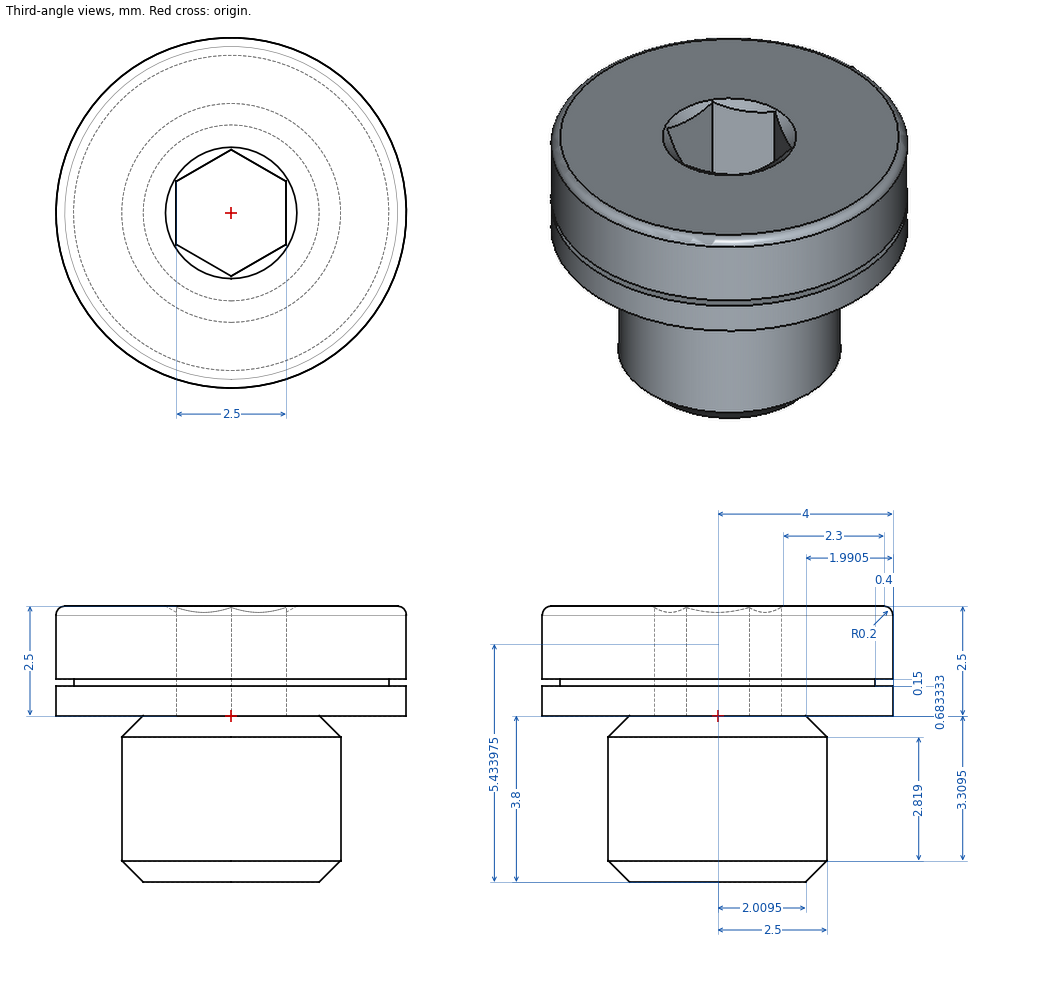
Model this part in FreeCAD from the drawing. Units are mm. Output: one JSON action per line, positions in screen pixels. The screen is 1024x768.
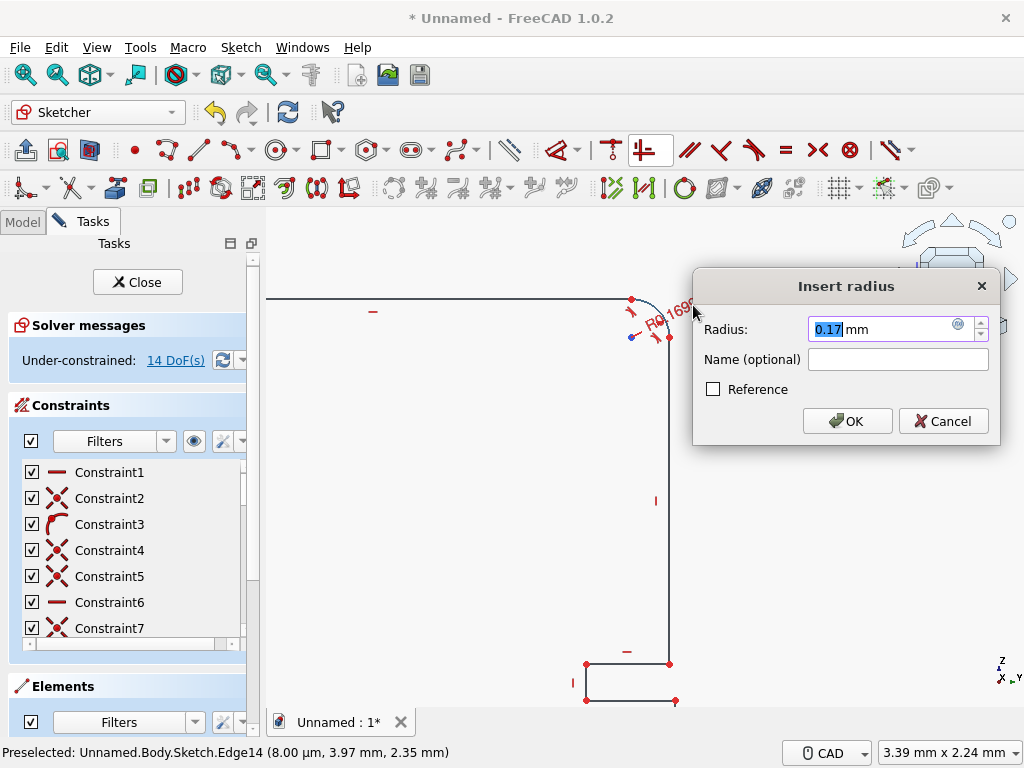
{"action": "type", "text": "0.2"}
{"action": "key", "text": "Return"}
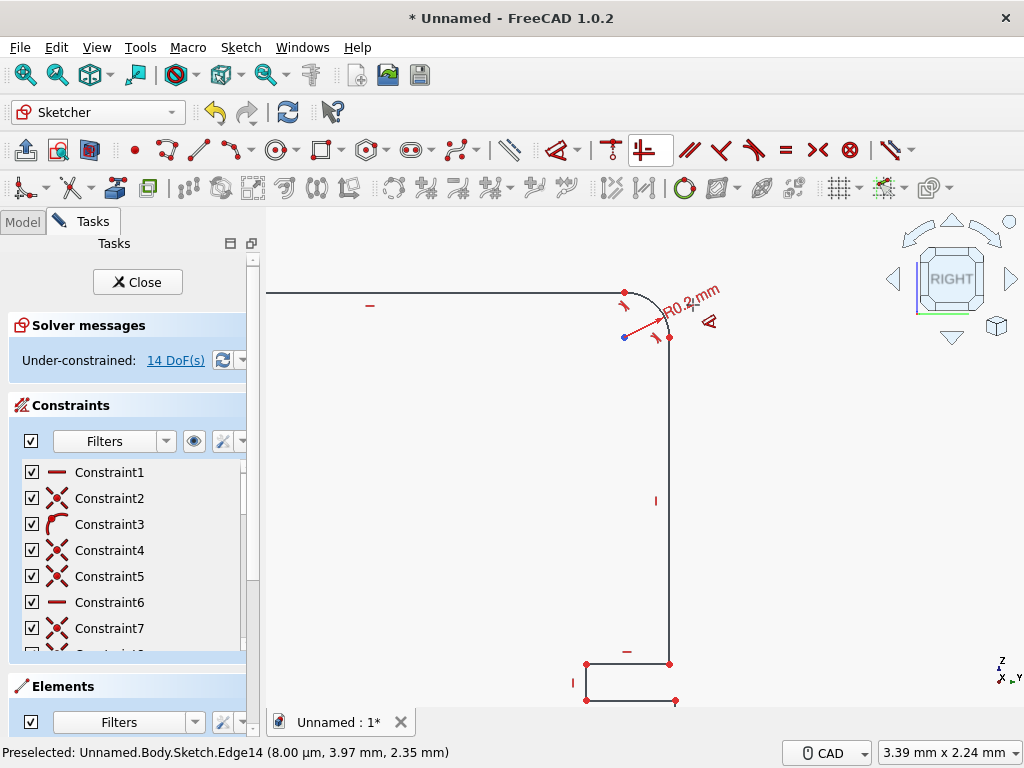
{"action": "scroll", "coordinate": [665, 321], "scroll_direction": "down", "scroll_amount": 8}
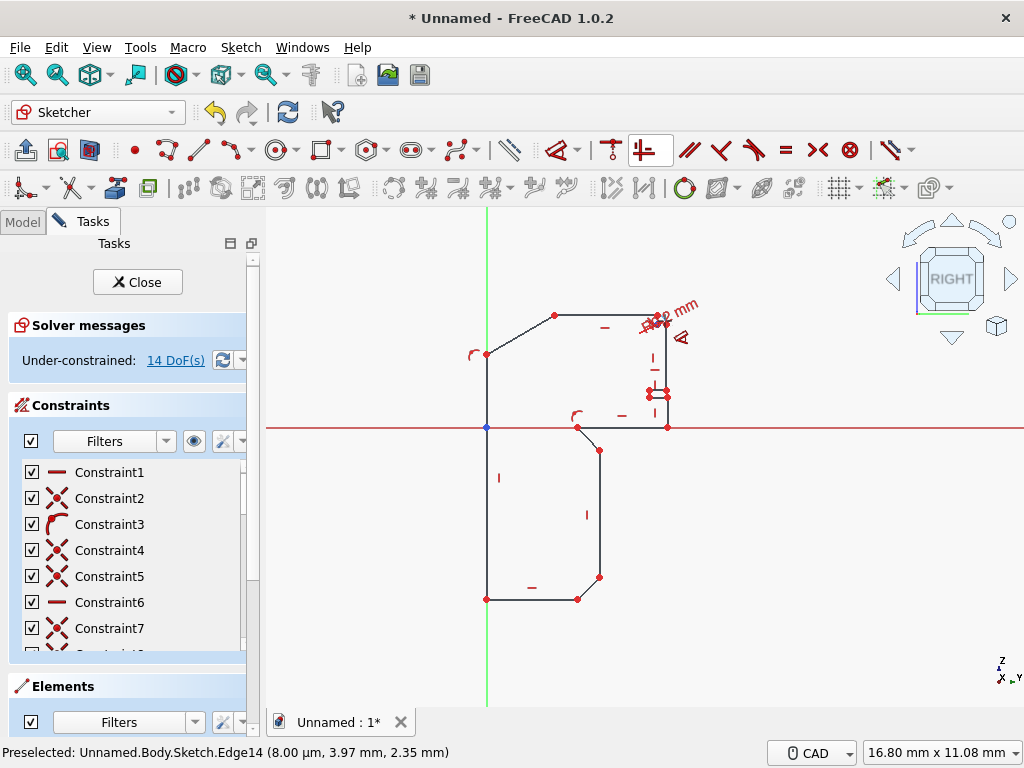
{"action": "left_click", "coordinate": [668, 428]}
{"action": "left_click", "coordinate": [577, 394]}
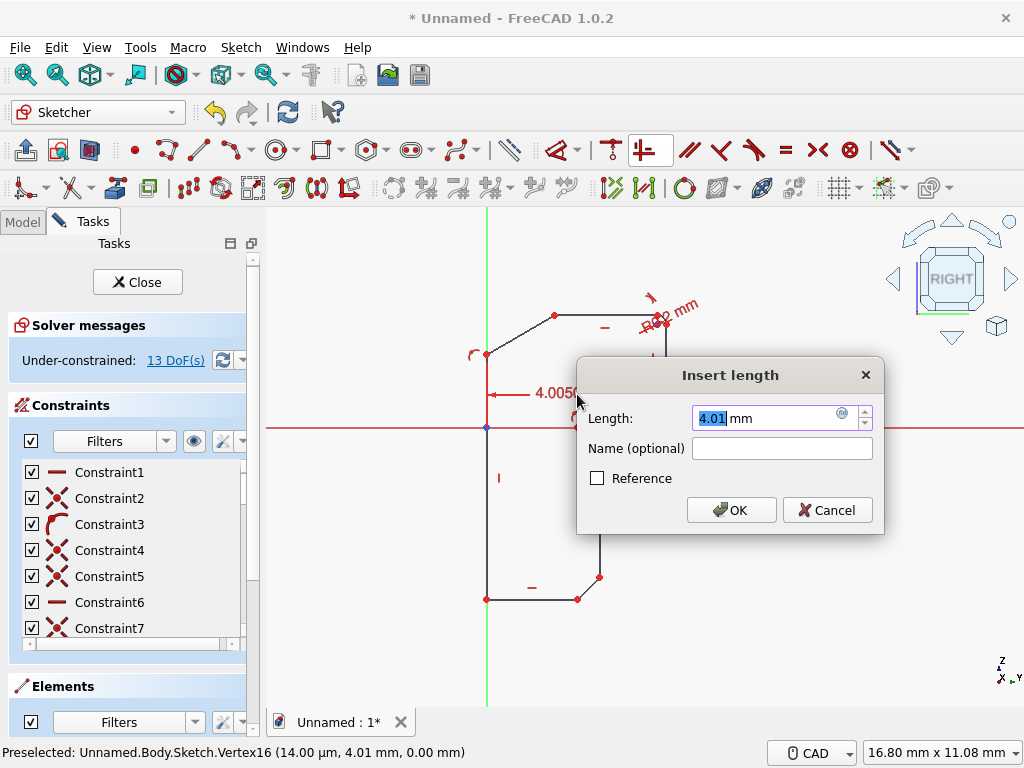
{"action": "type", "text": "4"}
{"action": "key", "text": "Return"}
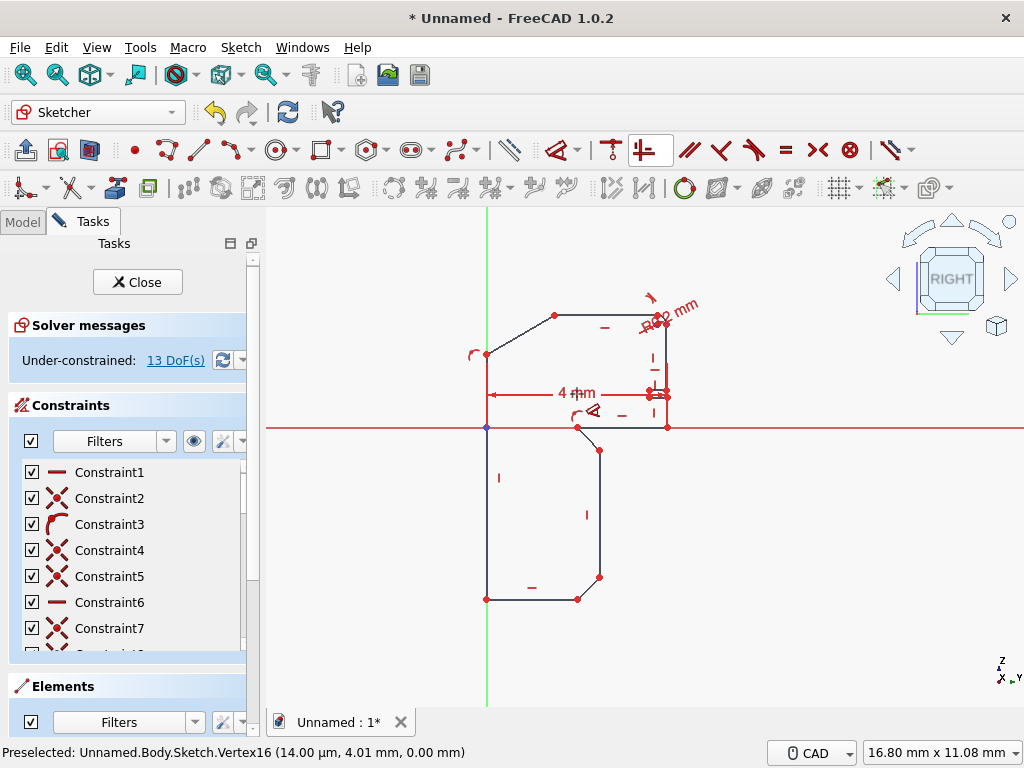
{"action": "scroll", "coordinate": [666, 390], "scroll_direction": "up", "scroll_amount": 3}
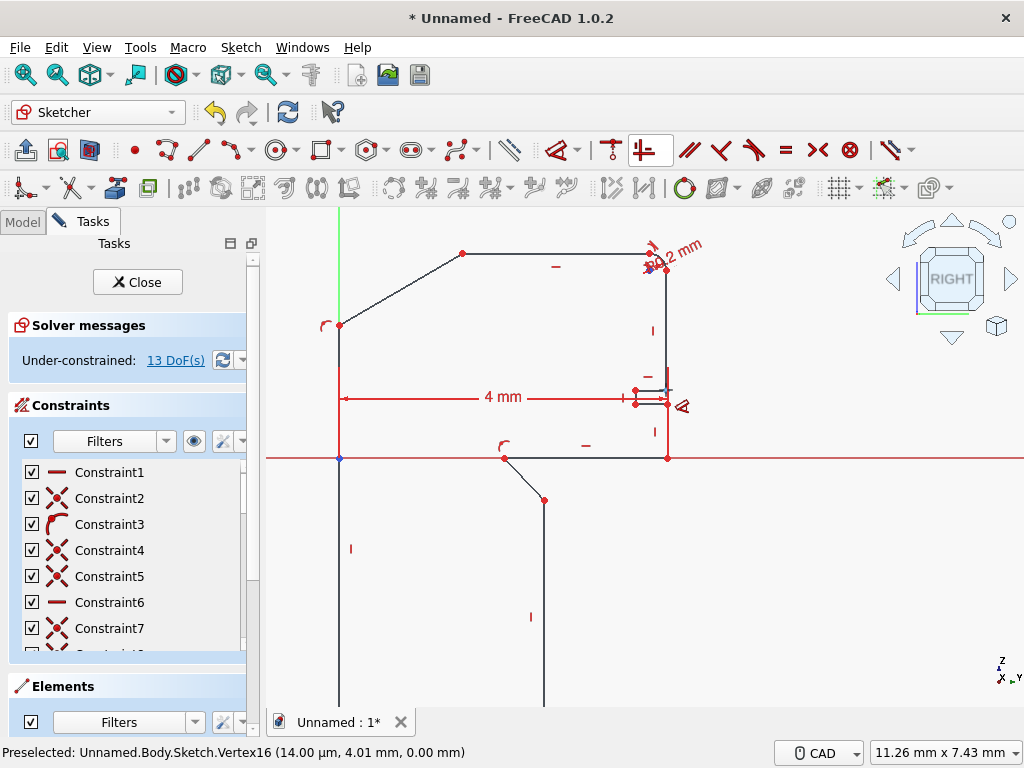
{"action": "left_click", "coordinate": [666, 391]}
{"action": "left_click", "coordinate": [503, 357]}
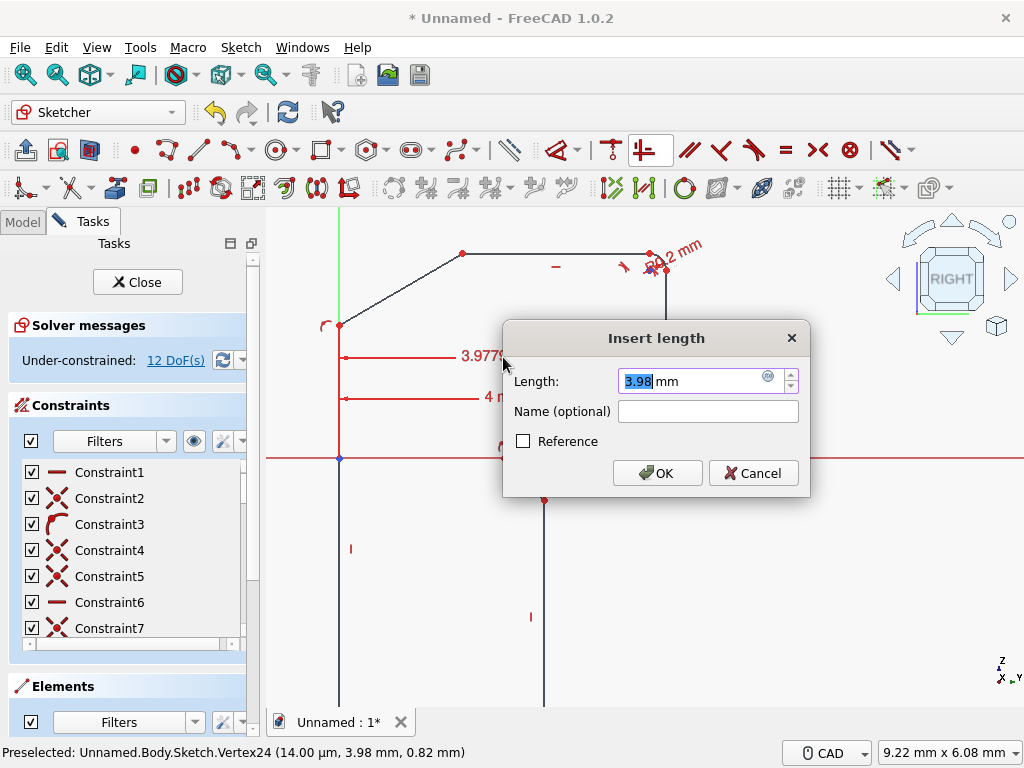
{"action": "type", "text": "4"}
{"action": "key", "text": "Return"}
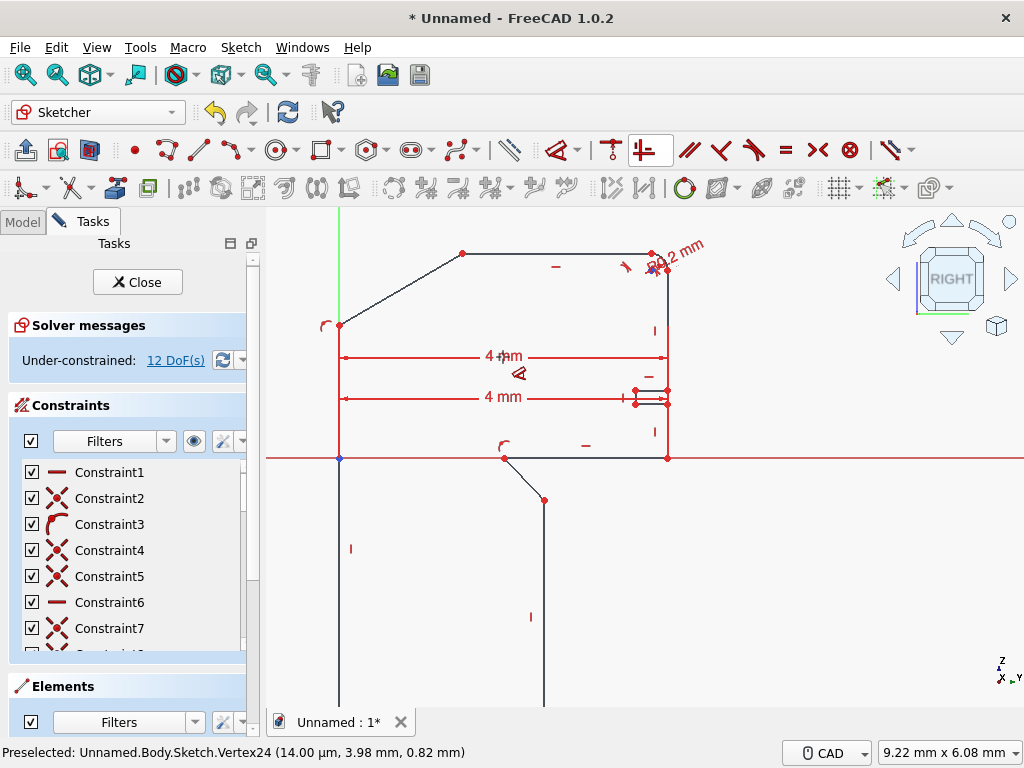
{"action": "left_click", "coordinate": [595, 254]}
{"action": "left_click", "coordinate": [557, 288]}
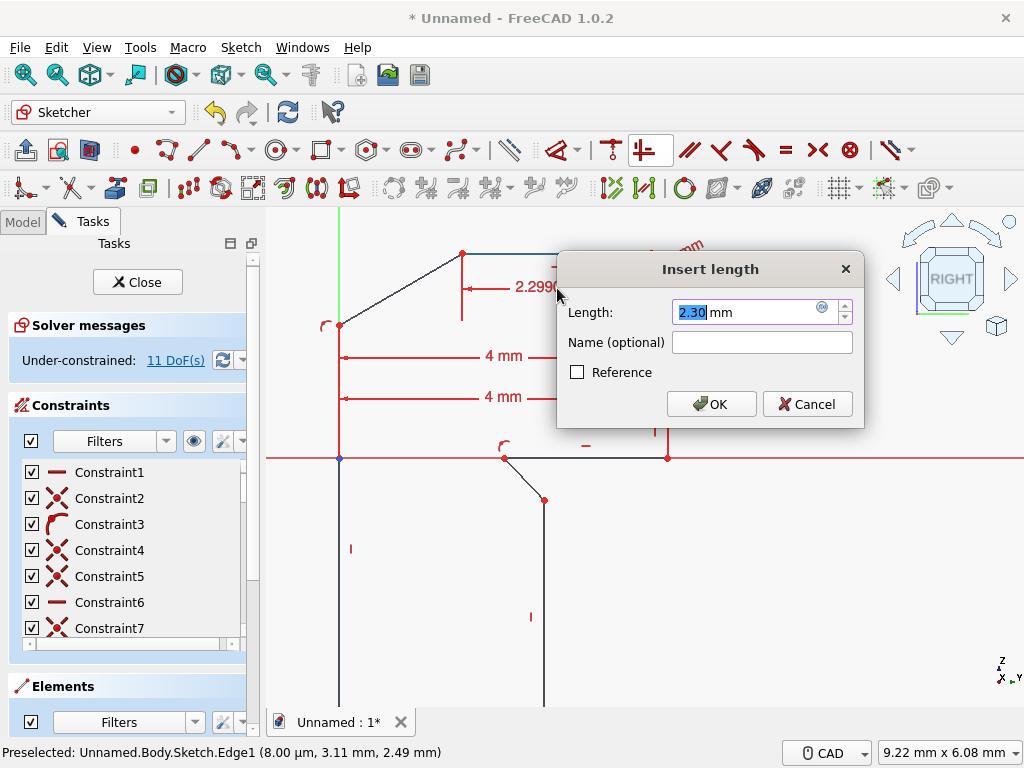
{"action": "type", "text": "2.3"}
{"action": "key", "text": "Return"}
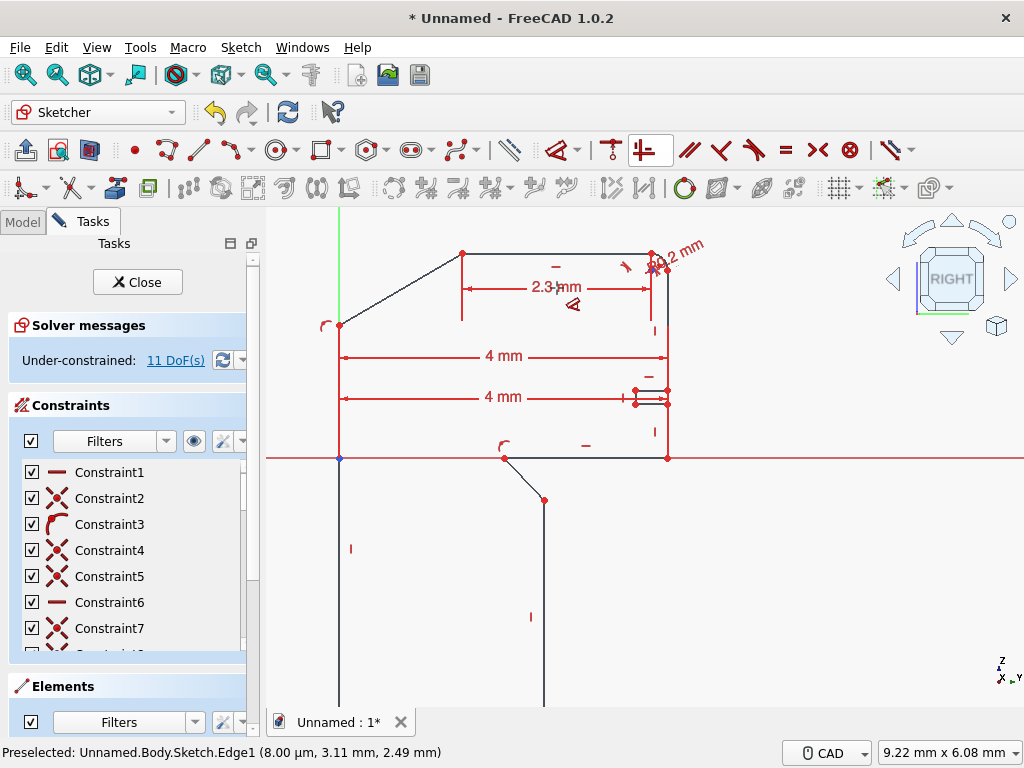
{"action": "scroll", "coordinate": [658, 404], "scroll_direction": "up", "scroll_amount": 2}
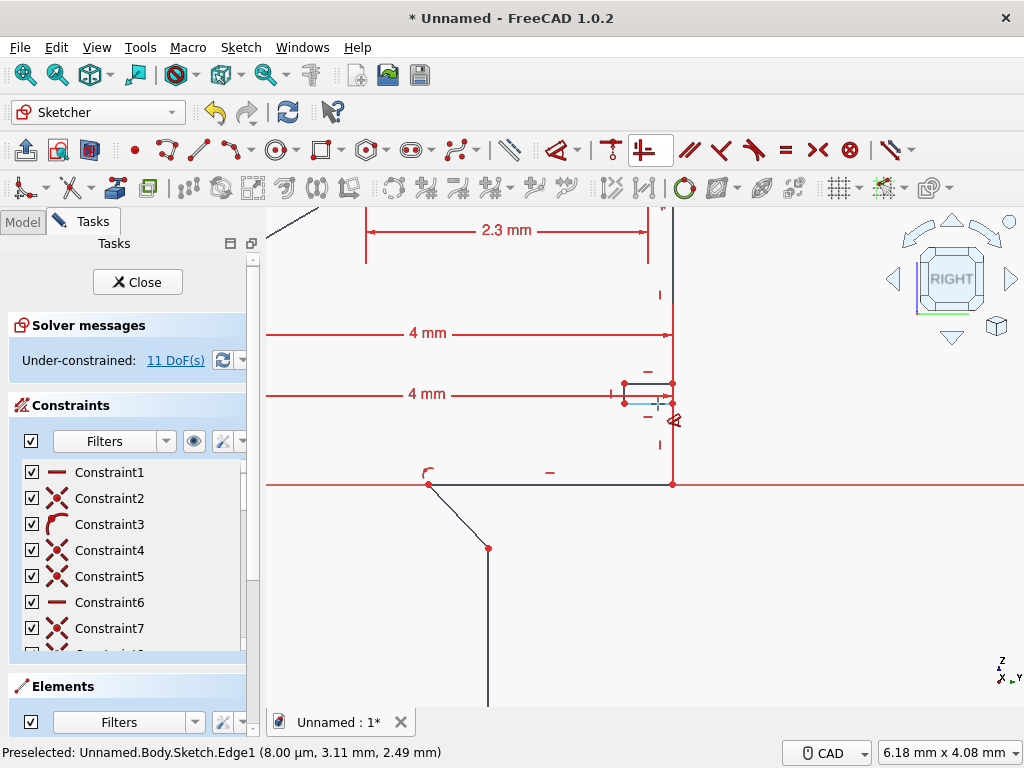
{"action": "left_click", "coordinate": [658, 404]}
{"action": "left_click", "coordinate": [648, 370]}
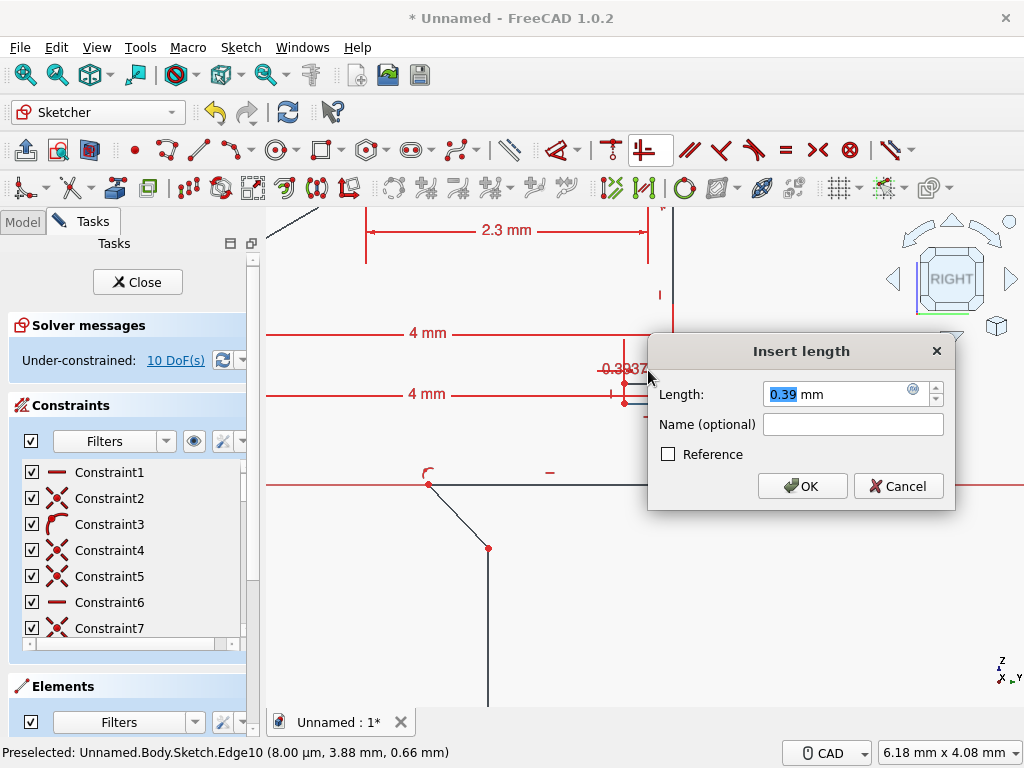
{"action": "type", "text": "0.4"}
{"action": "key", "text": "Return"}